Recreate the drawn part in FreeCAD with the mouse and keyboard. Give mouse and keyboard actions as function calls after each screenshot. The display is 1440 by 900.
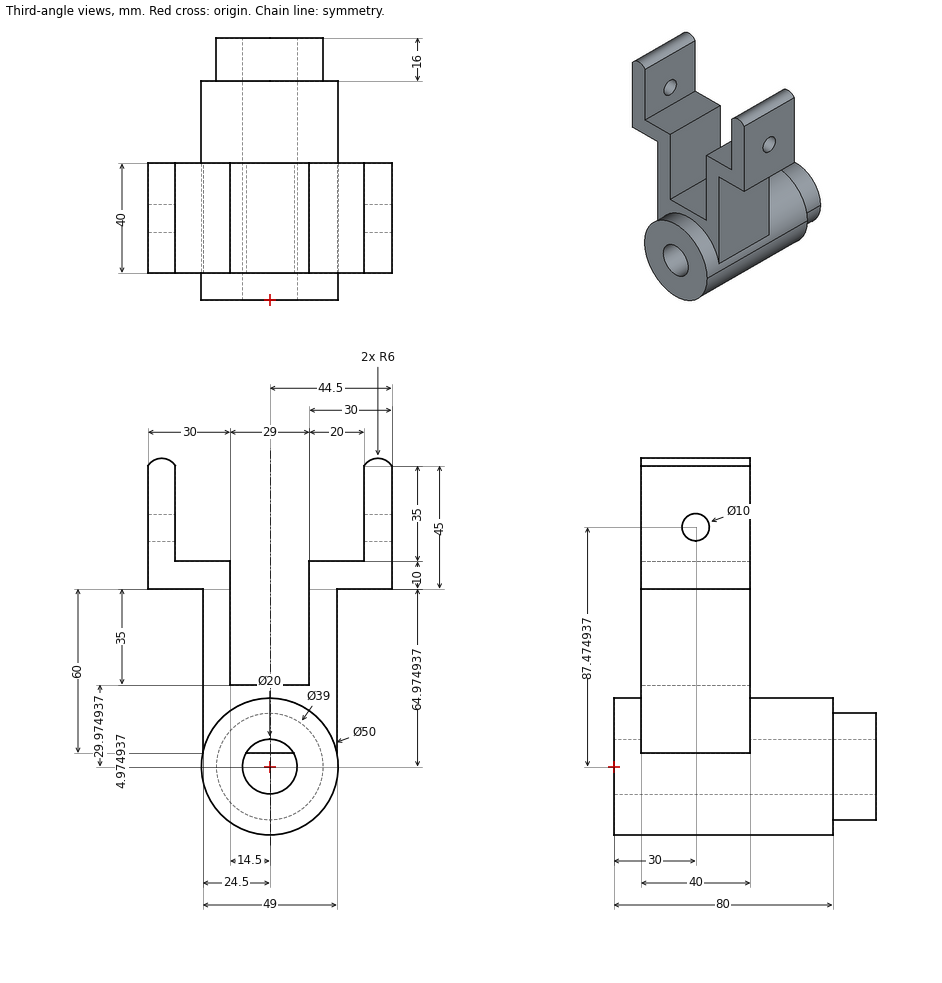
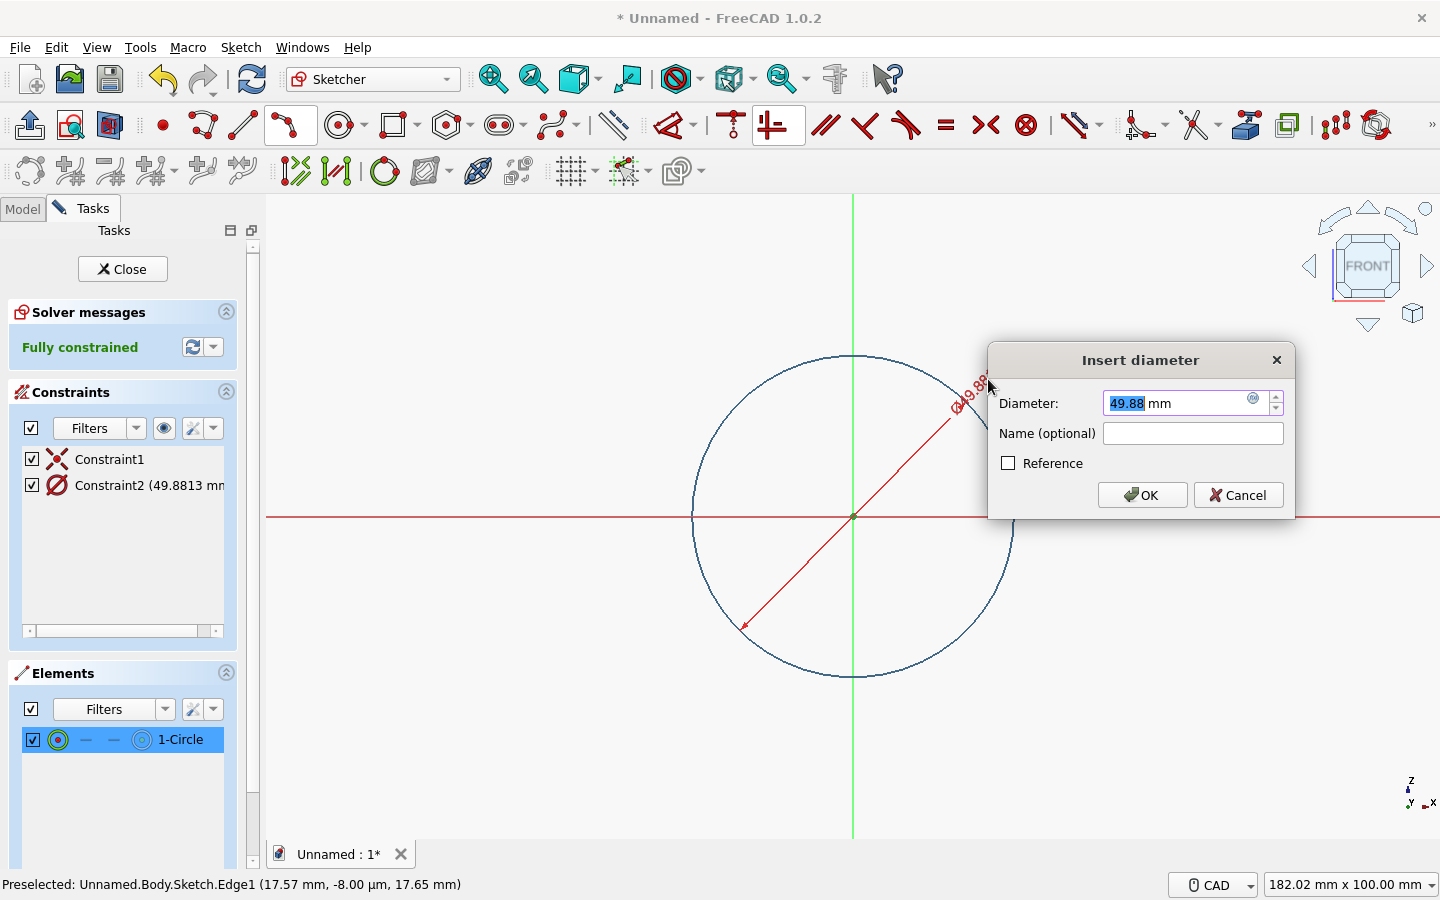
text(50)
key(Return)
key(Escape)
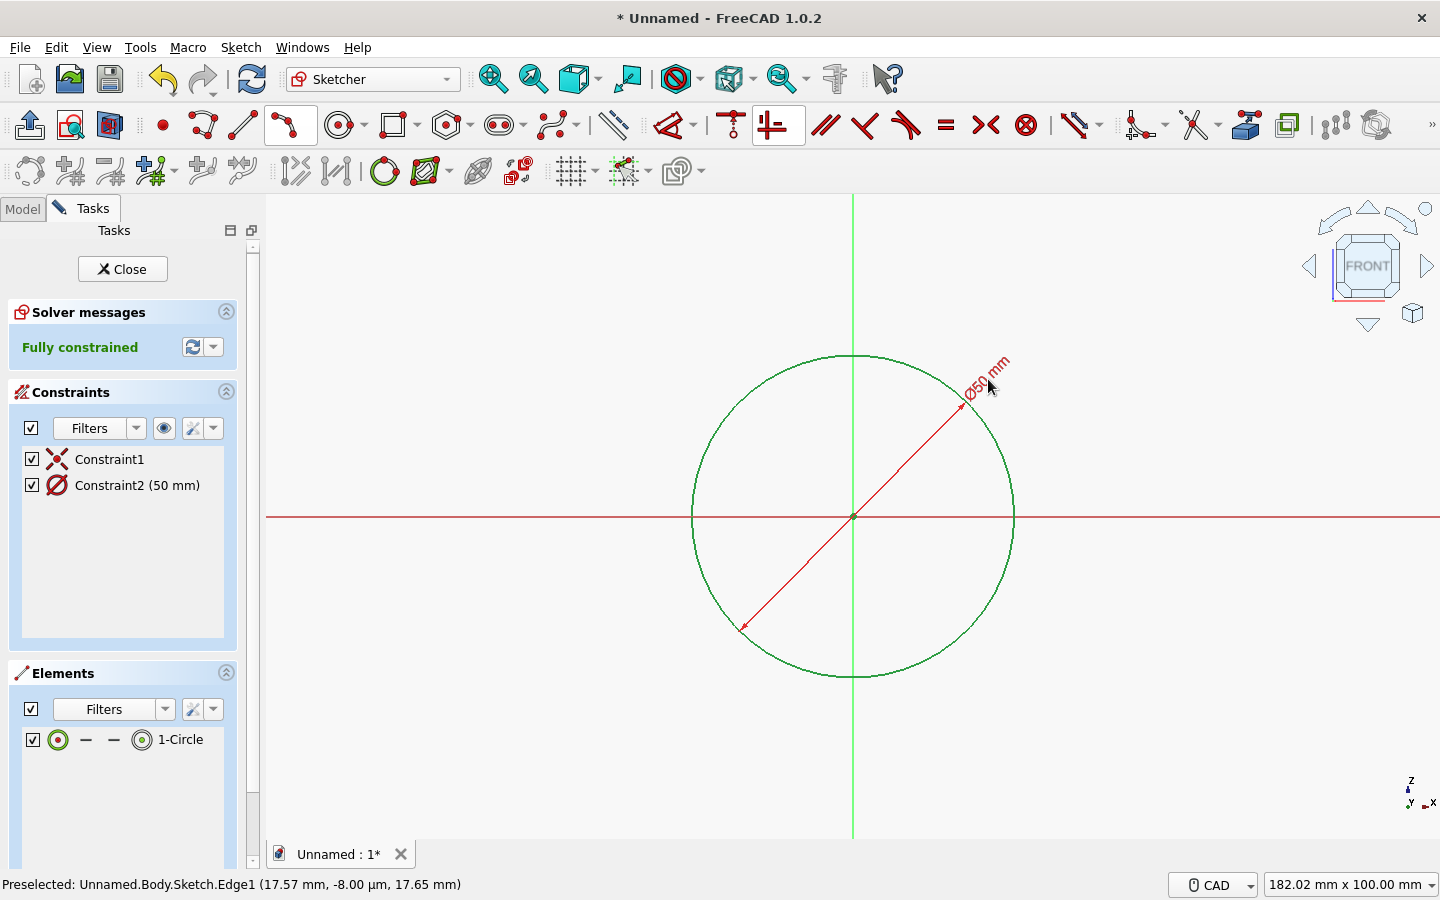
click(123, 269)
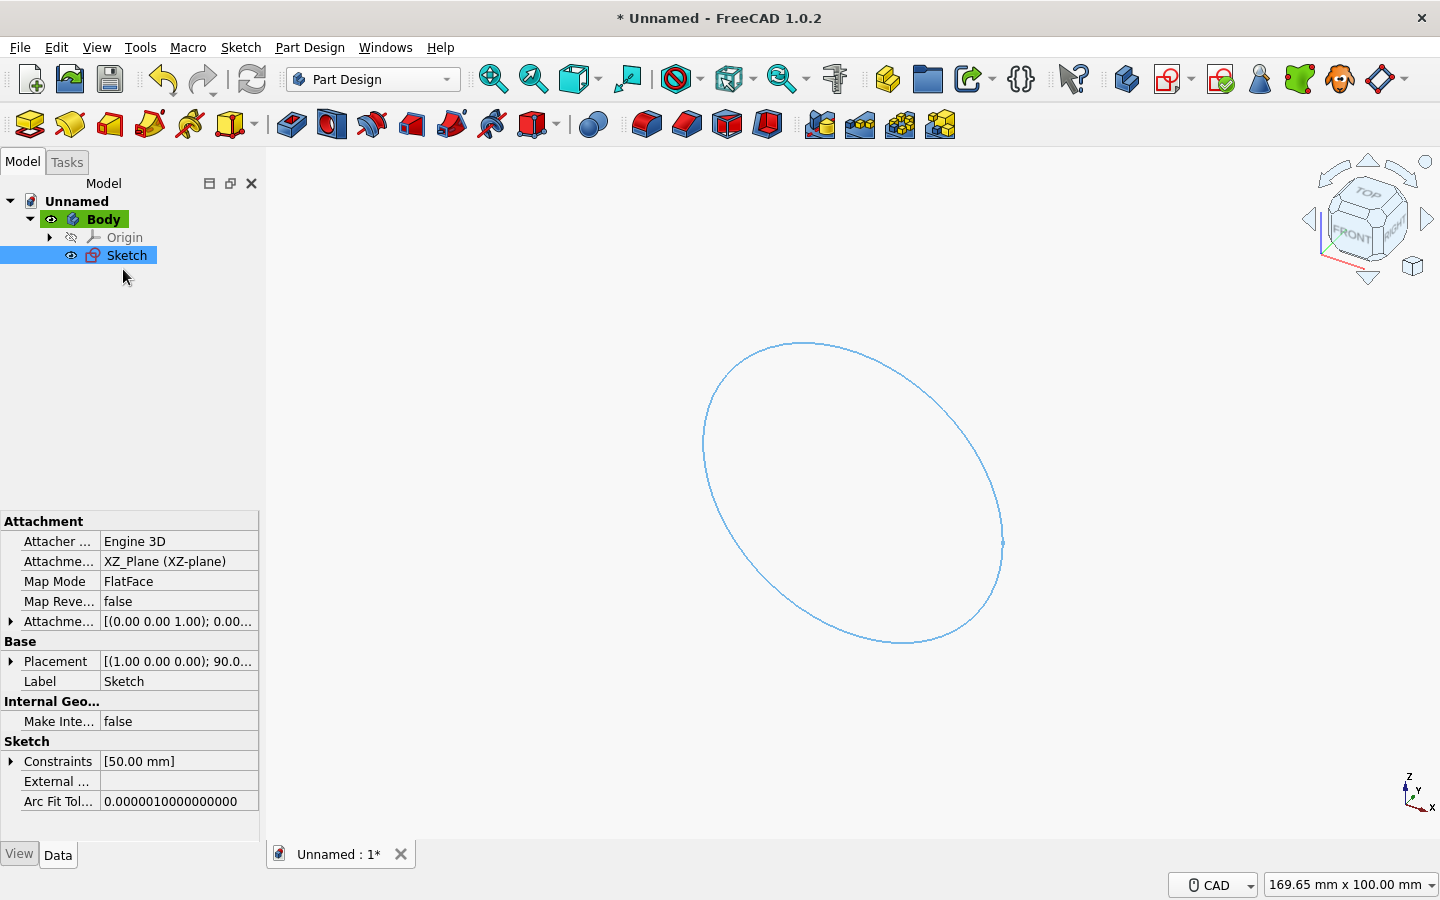
click(30, 124)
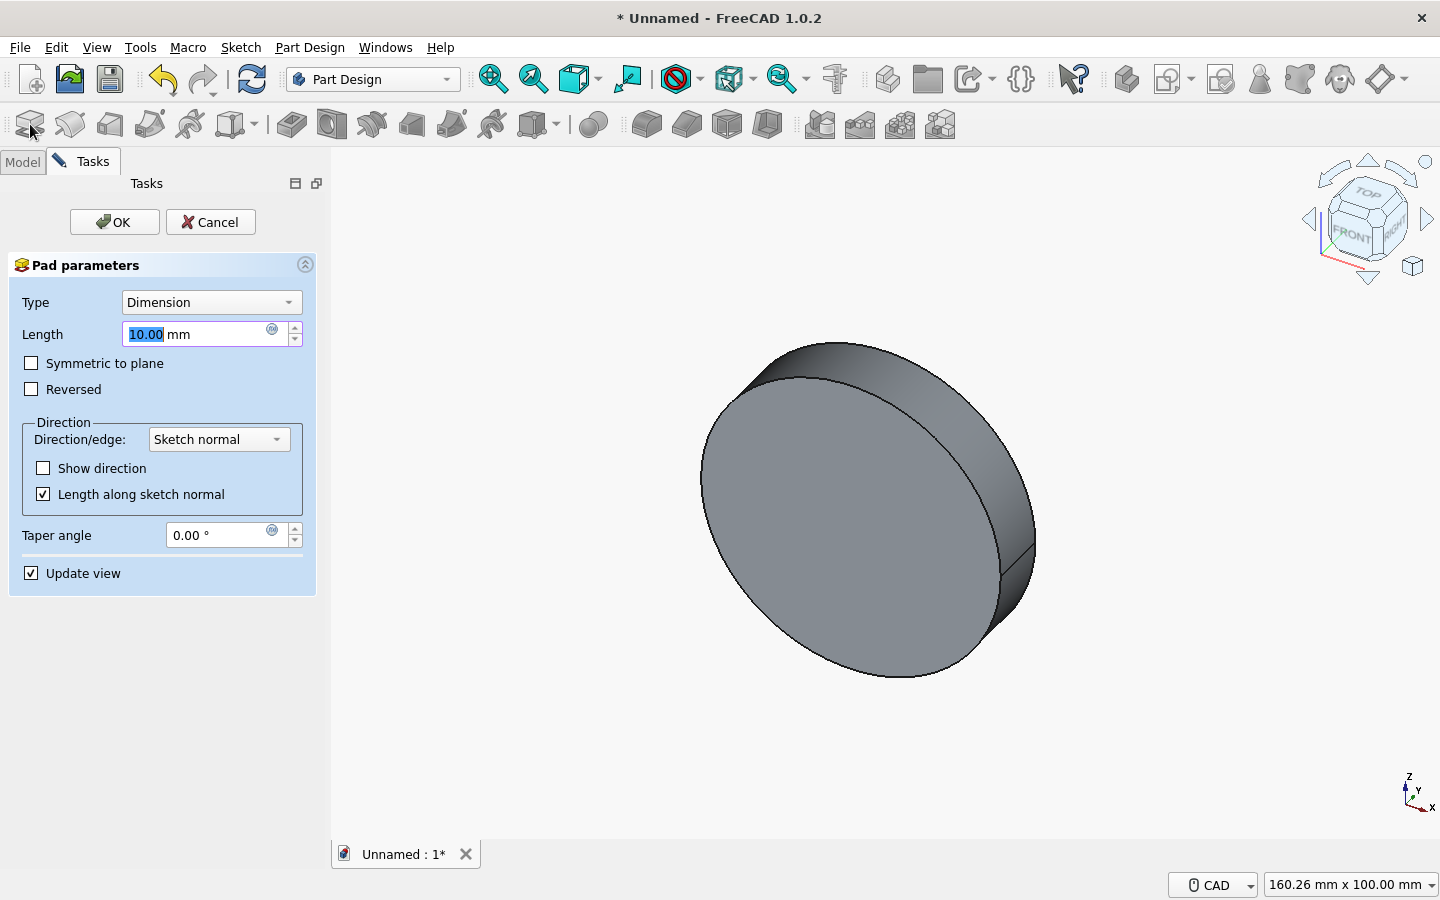
text(80)
key(Tab)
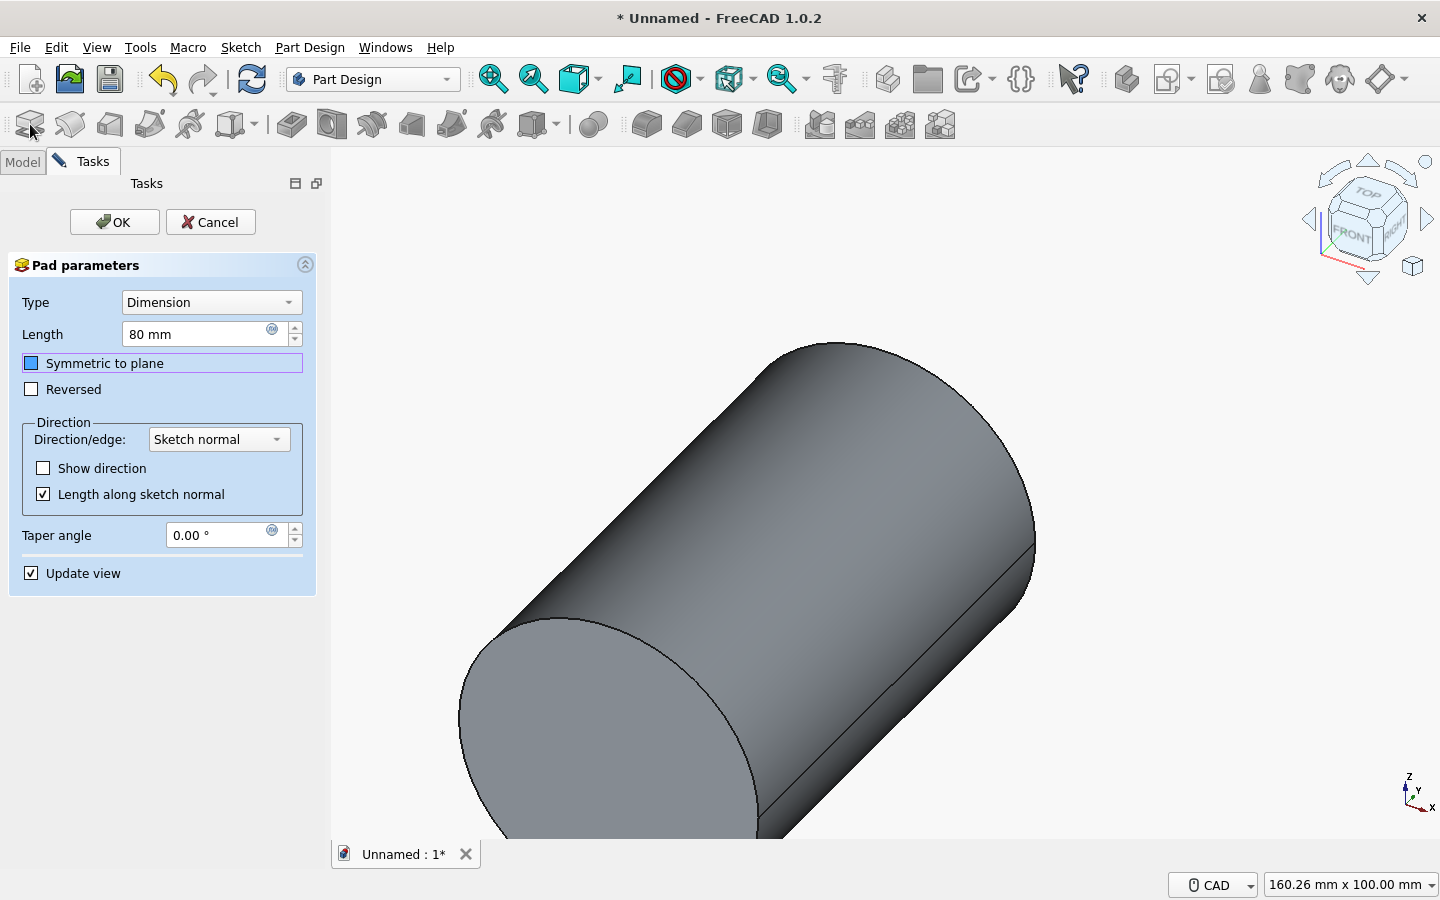
click(30, 389)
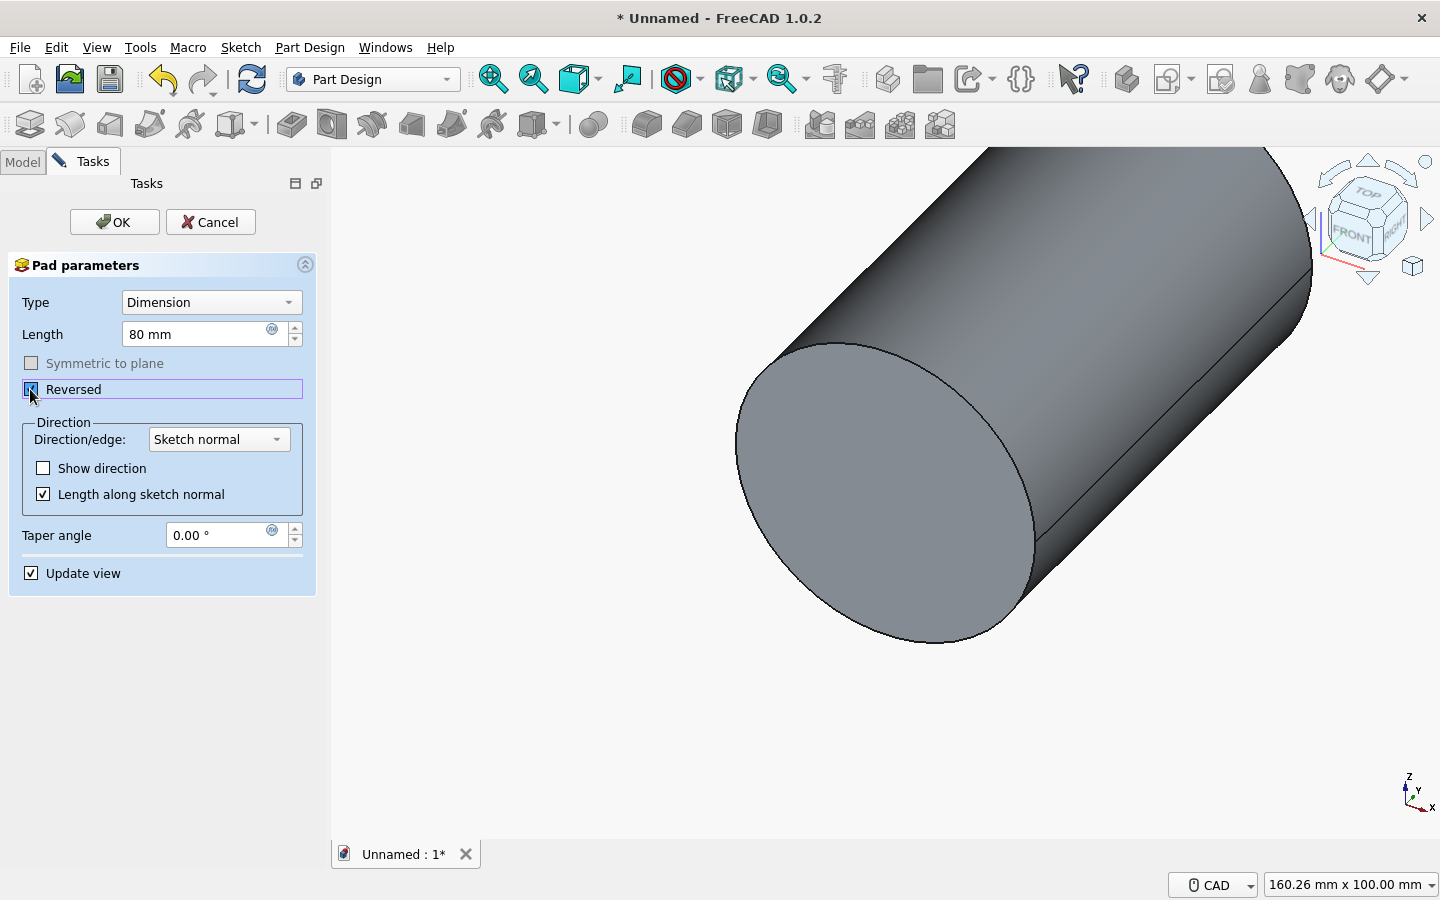
click(115, 222)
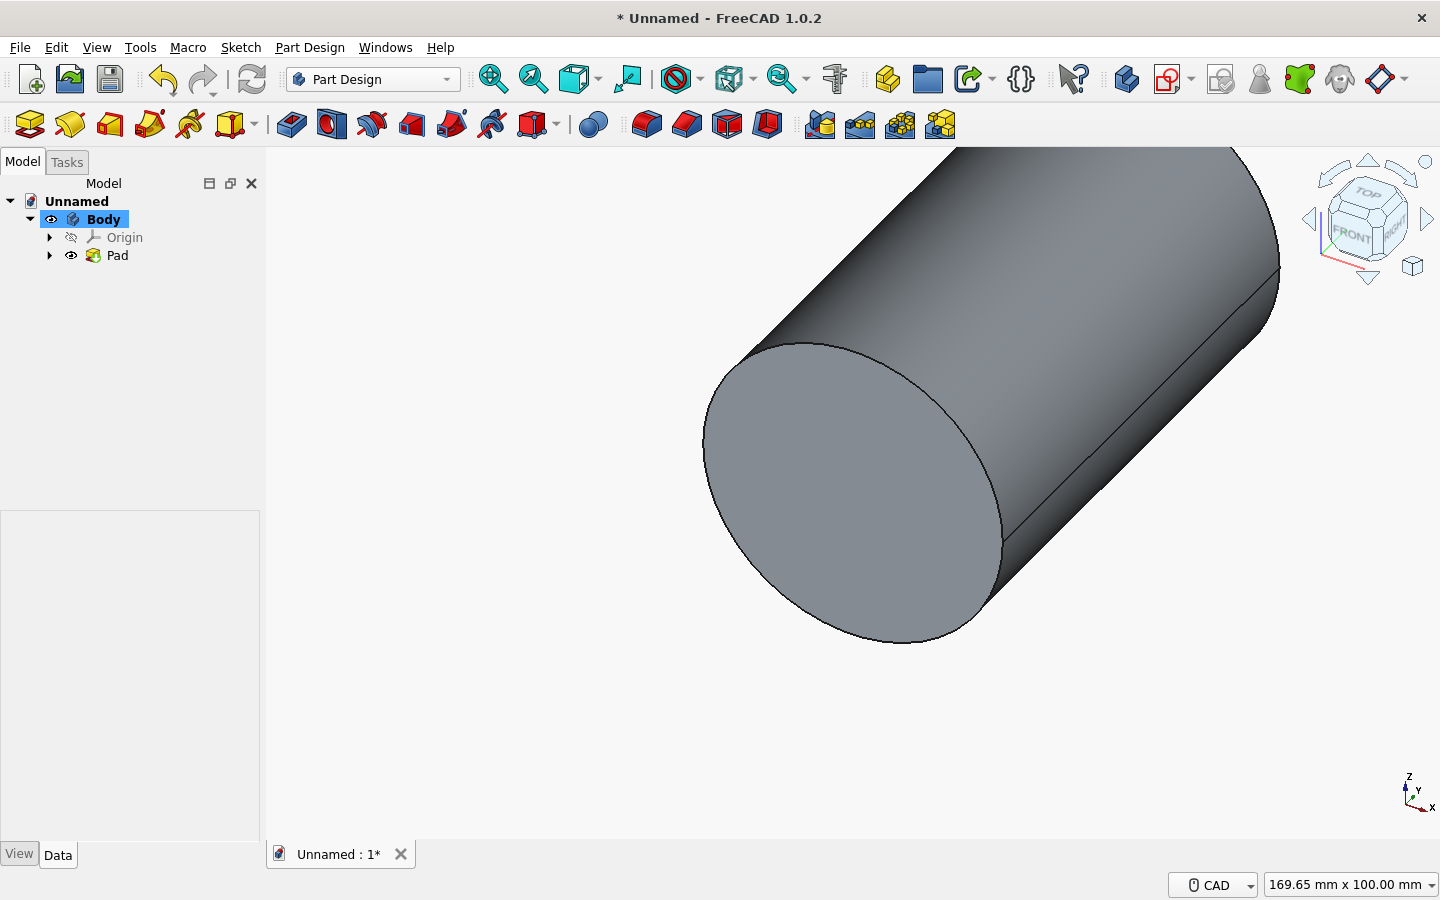
key(v)
key(f)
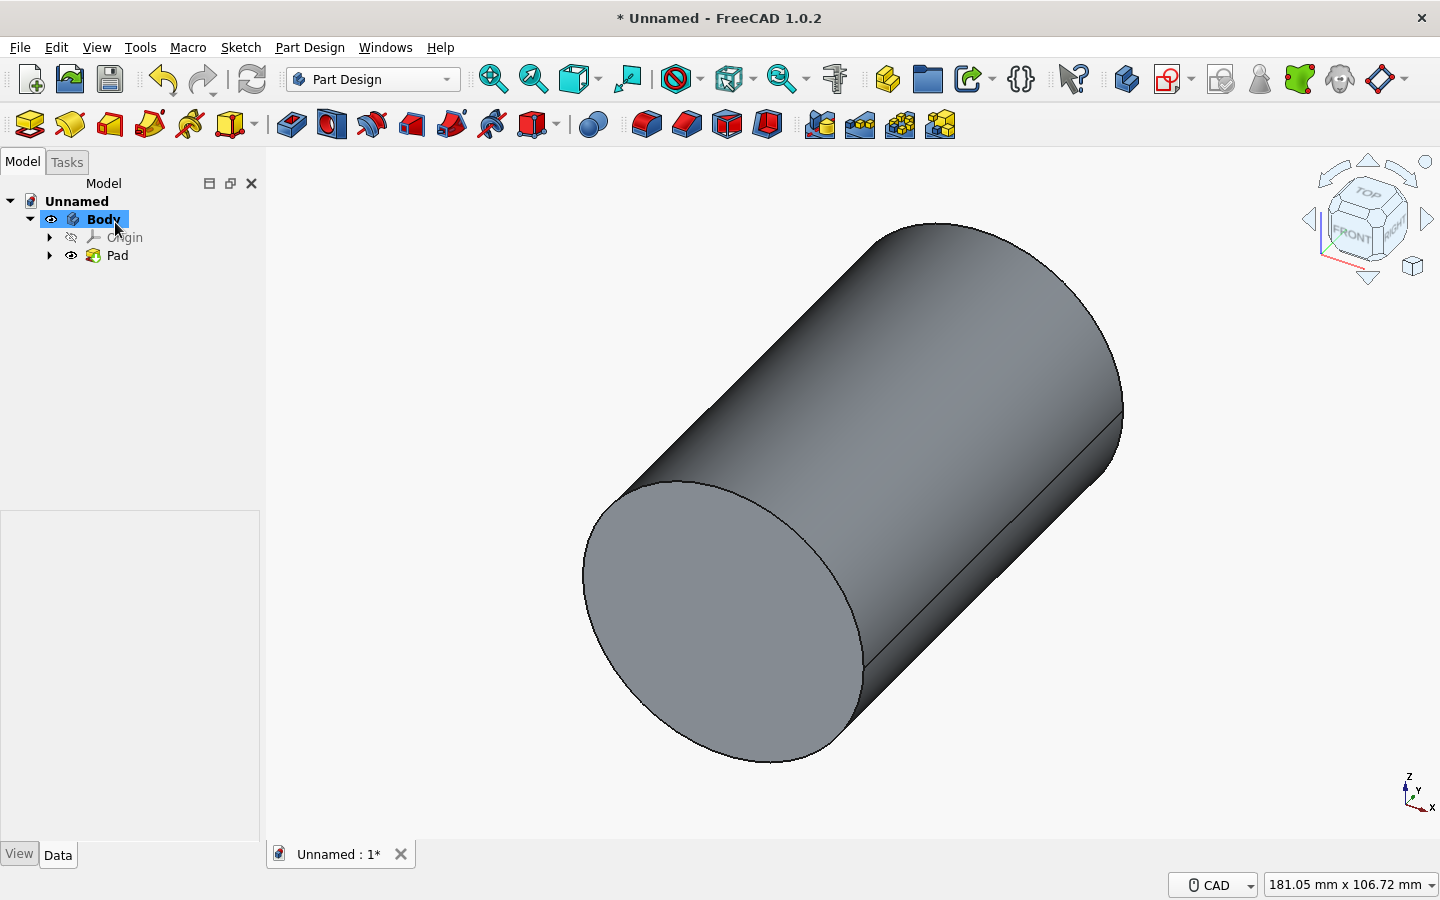
key(4)